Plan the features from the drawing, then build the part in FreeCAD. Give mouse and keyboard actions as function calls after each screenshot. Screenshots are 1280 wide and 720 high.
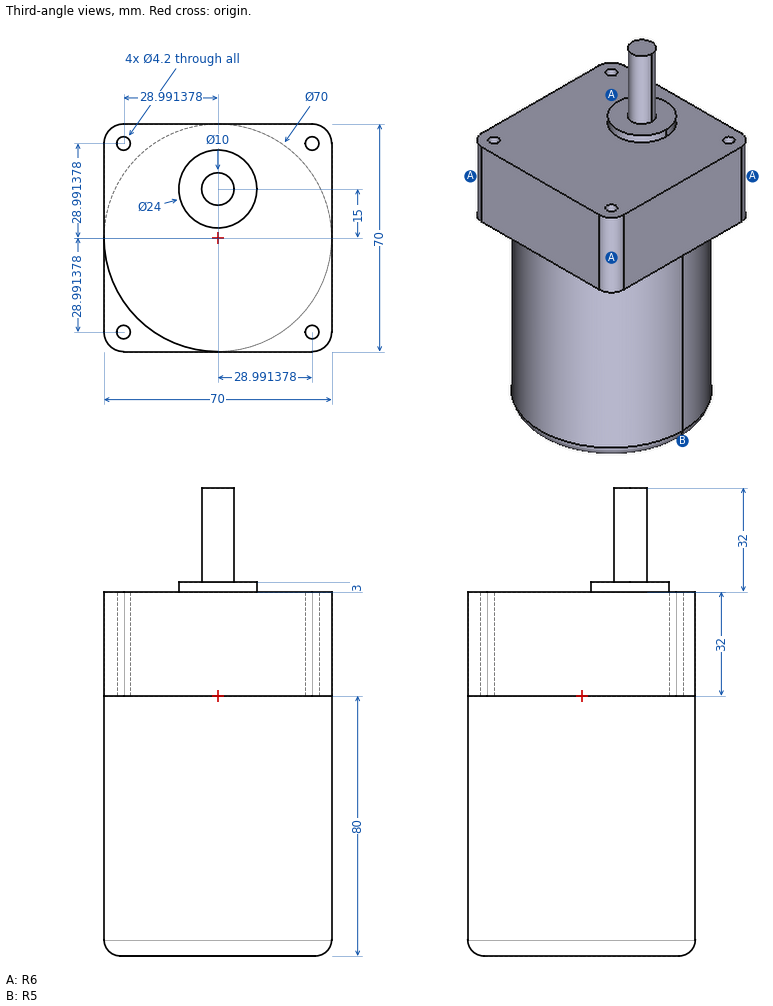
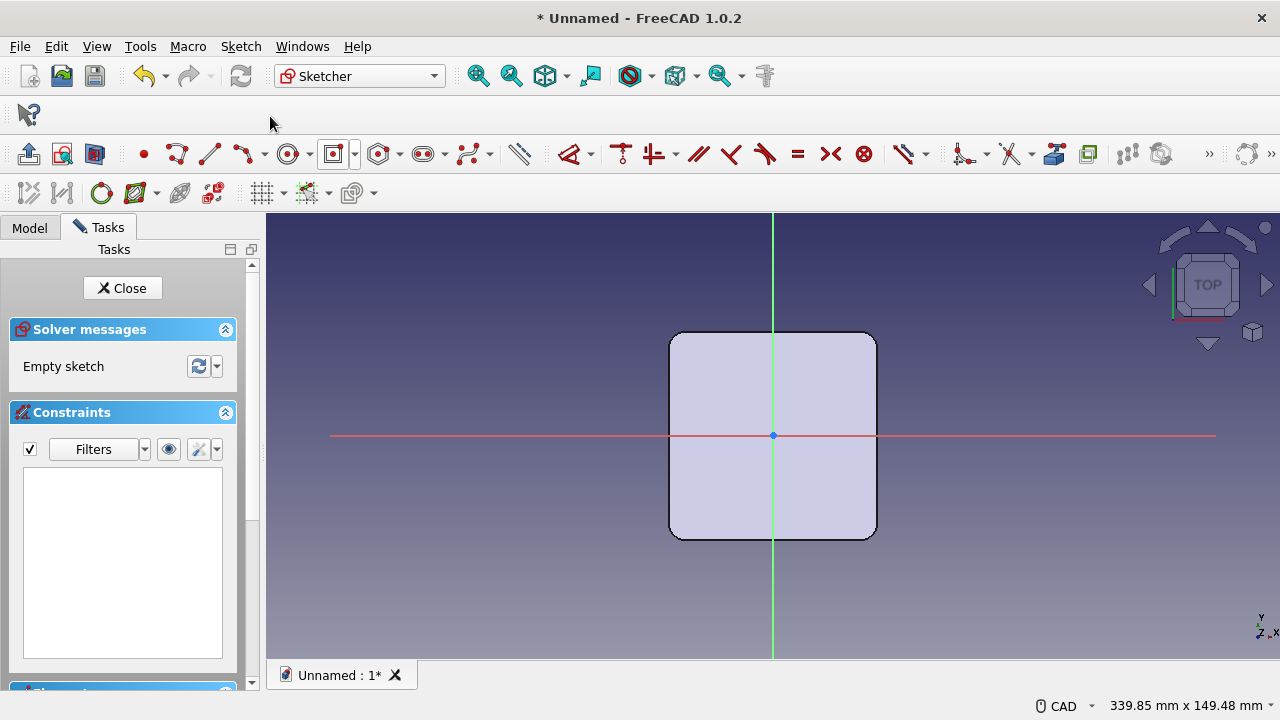
scroll(790, 399, up, 8)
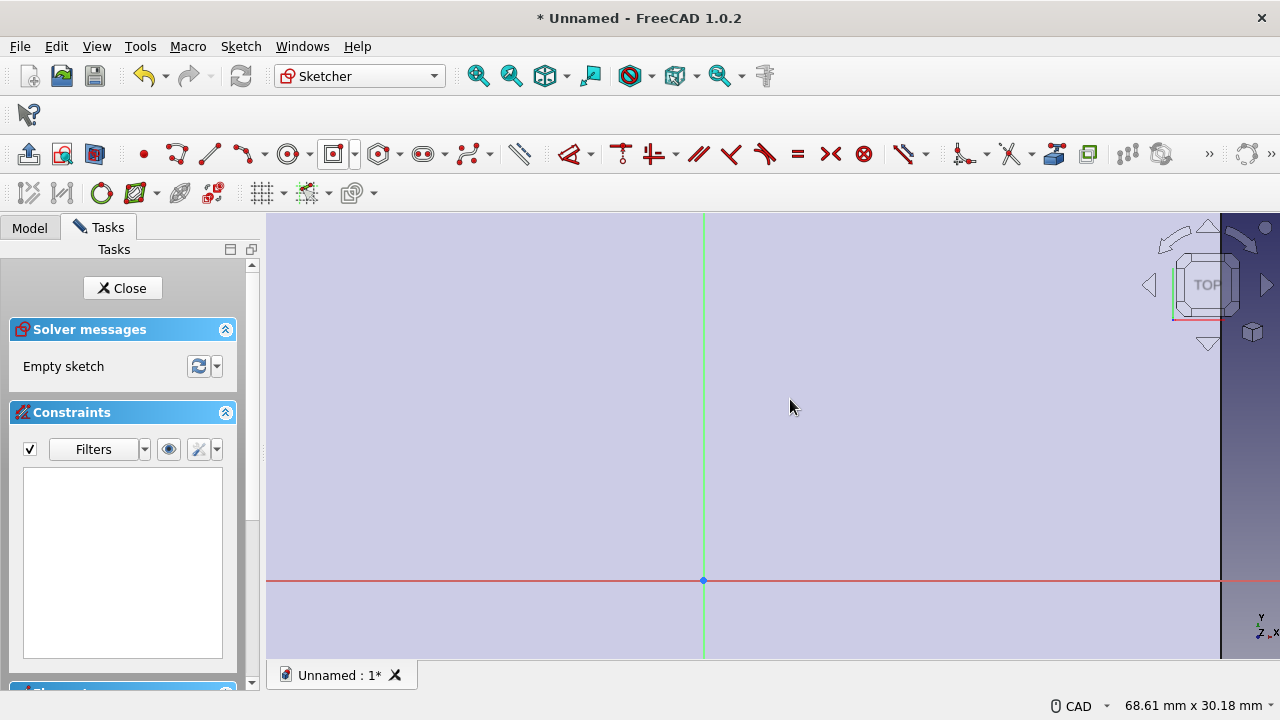
click(288, 154)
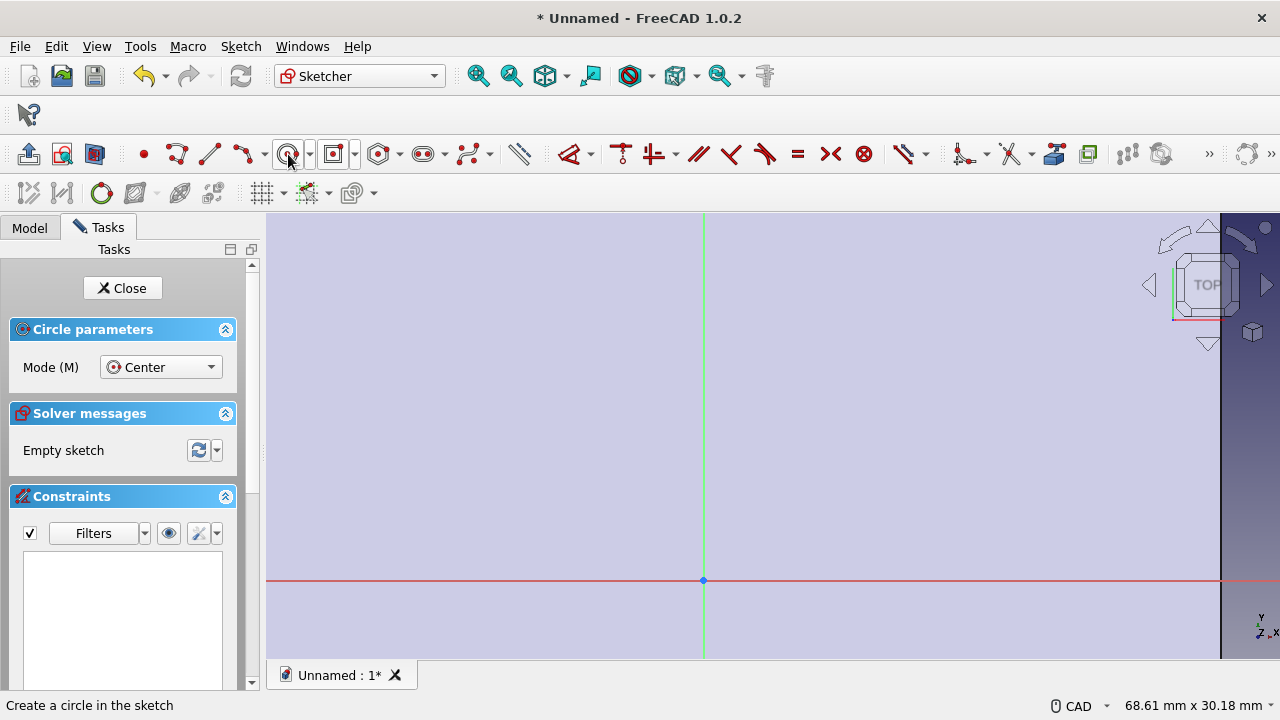
click(704, 359)
move(756, 307)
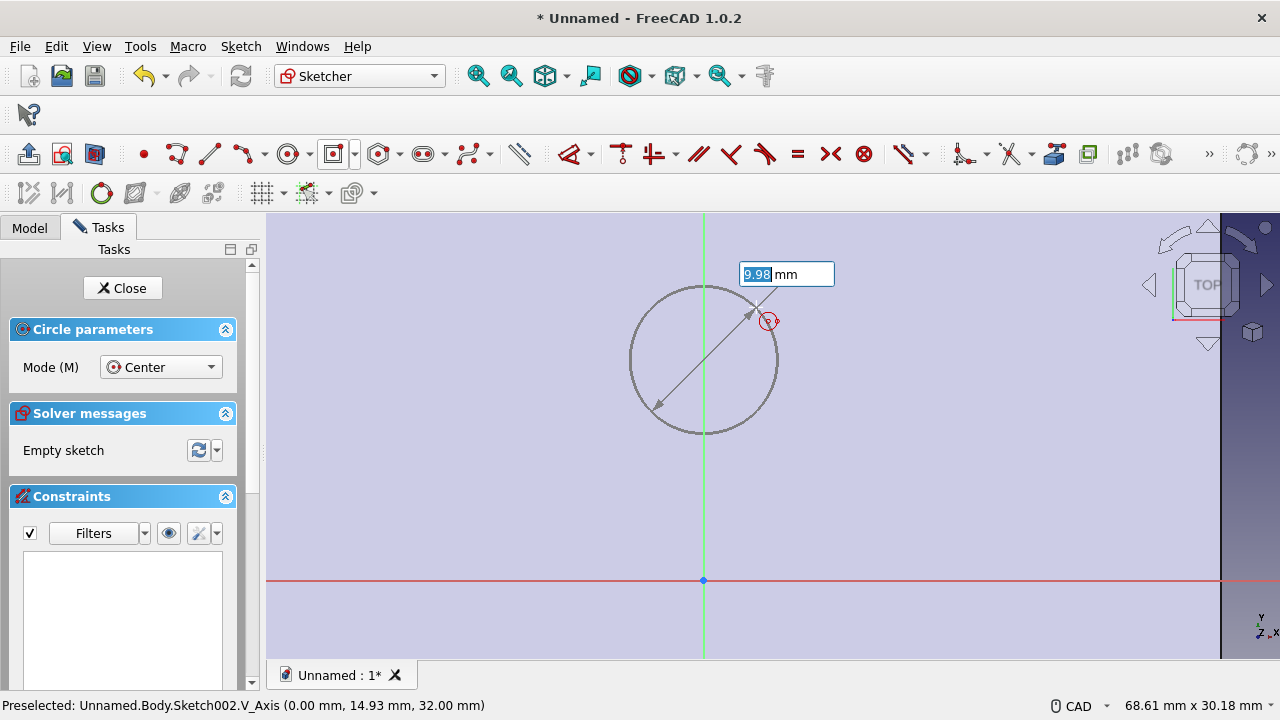
text(10)
key(Return)
key(Escape)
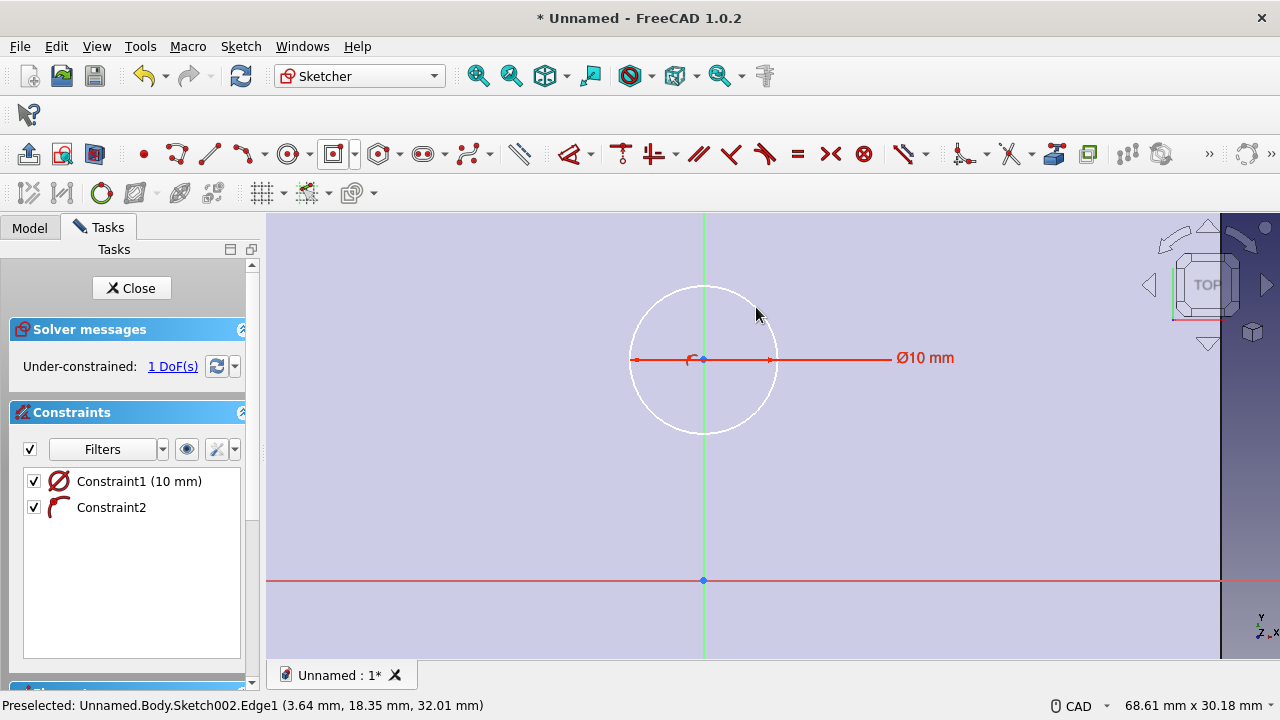
key(d)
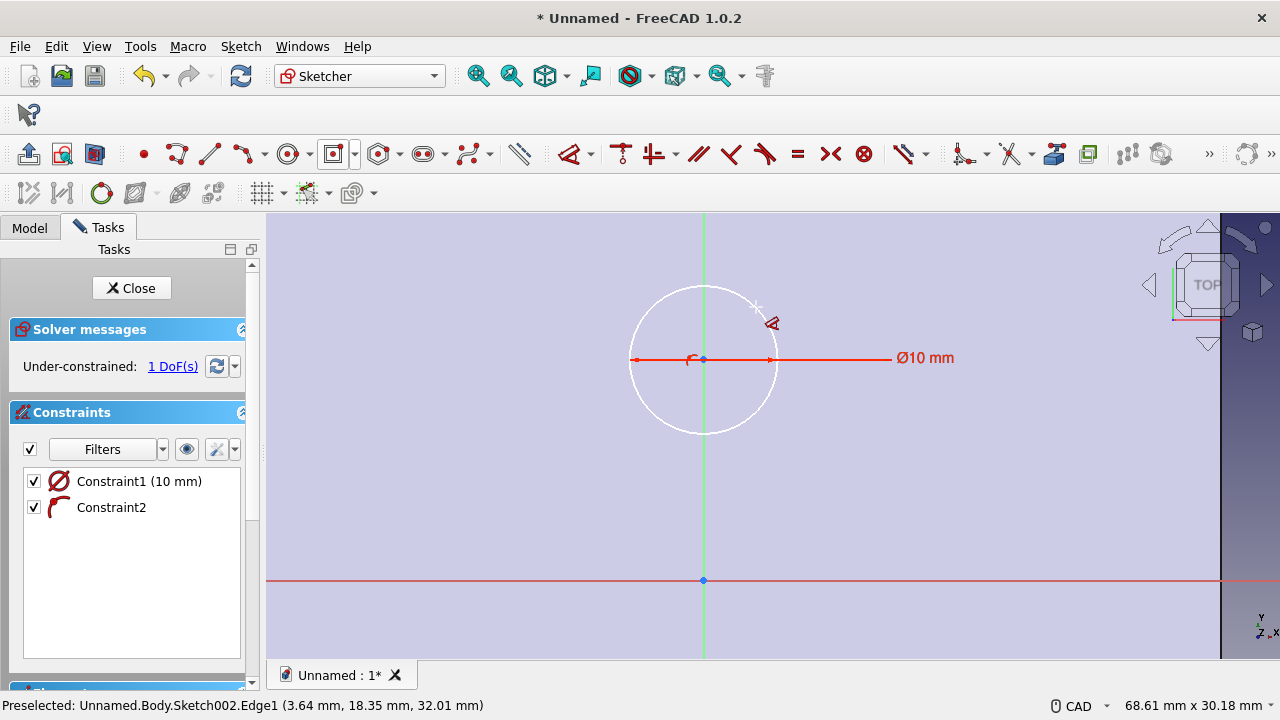
click(704, 360)
click(738, 470)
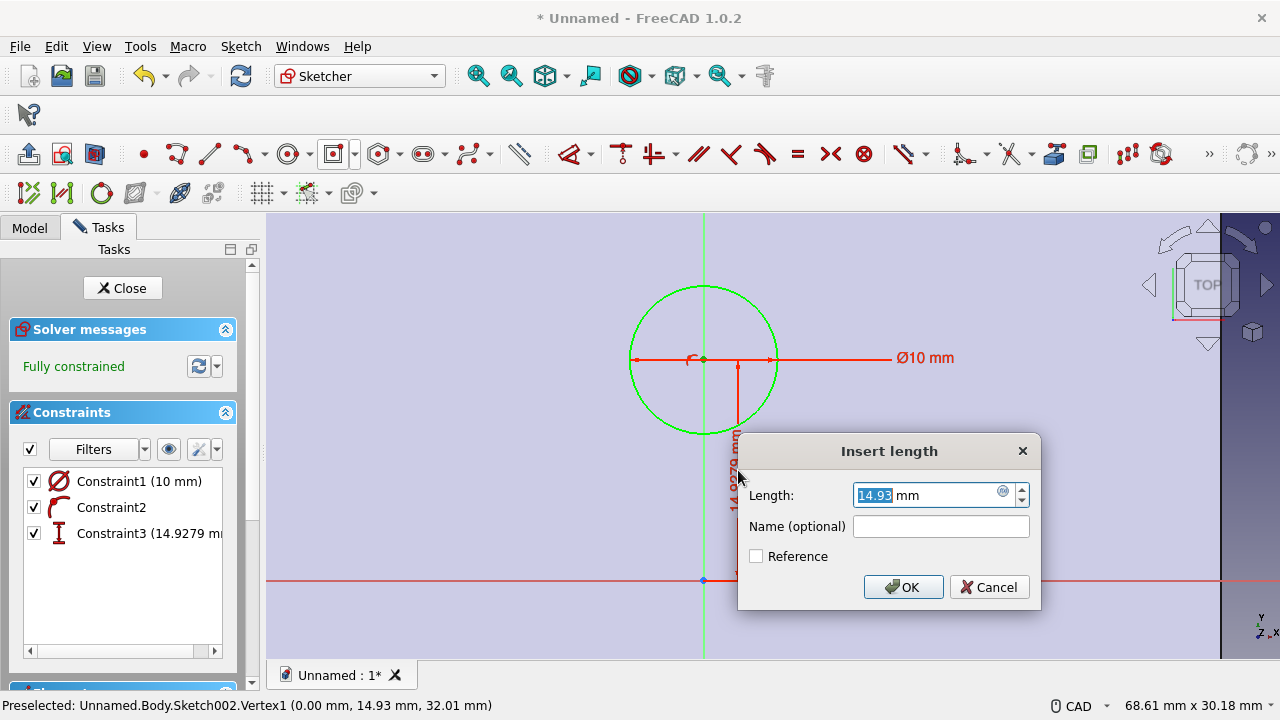
text(15)
key(Return)
key(Escape)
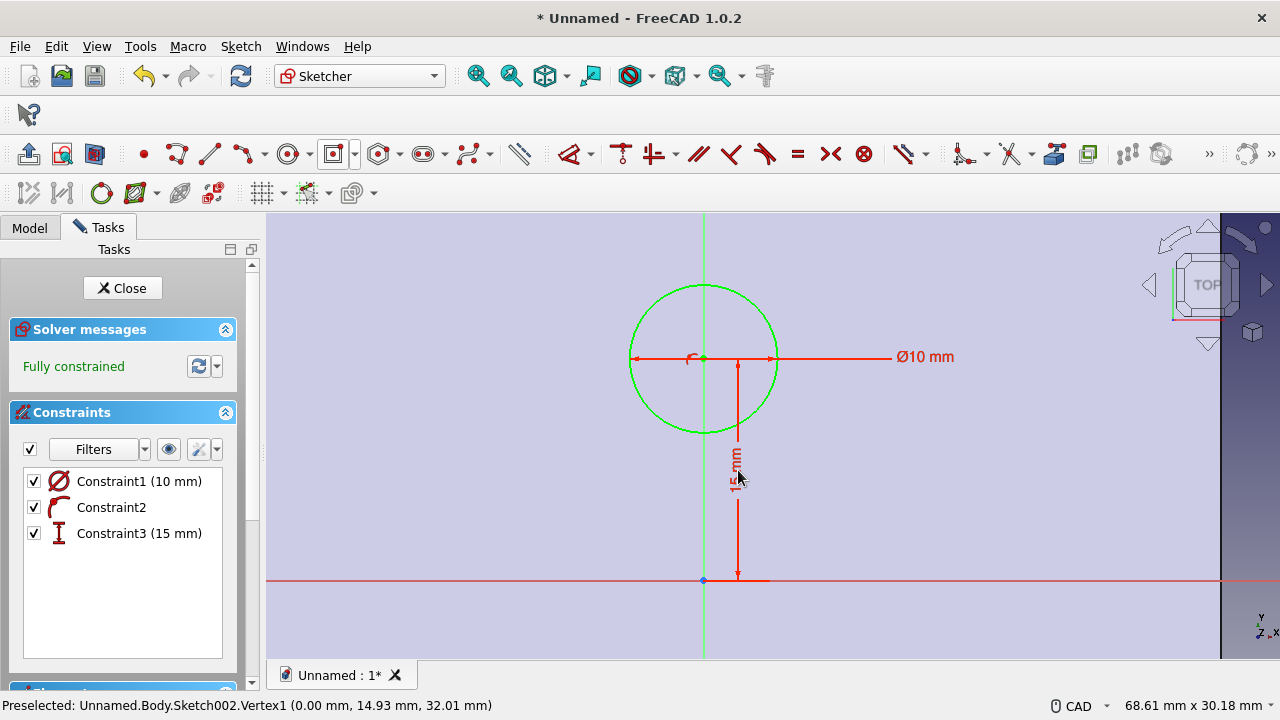
click(123, 288)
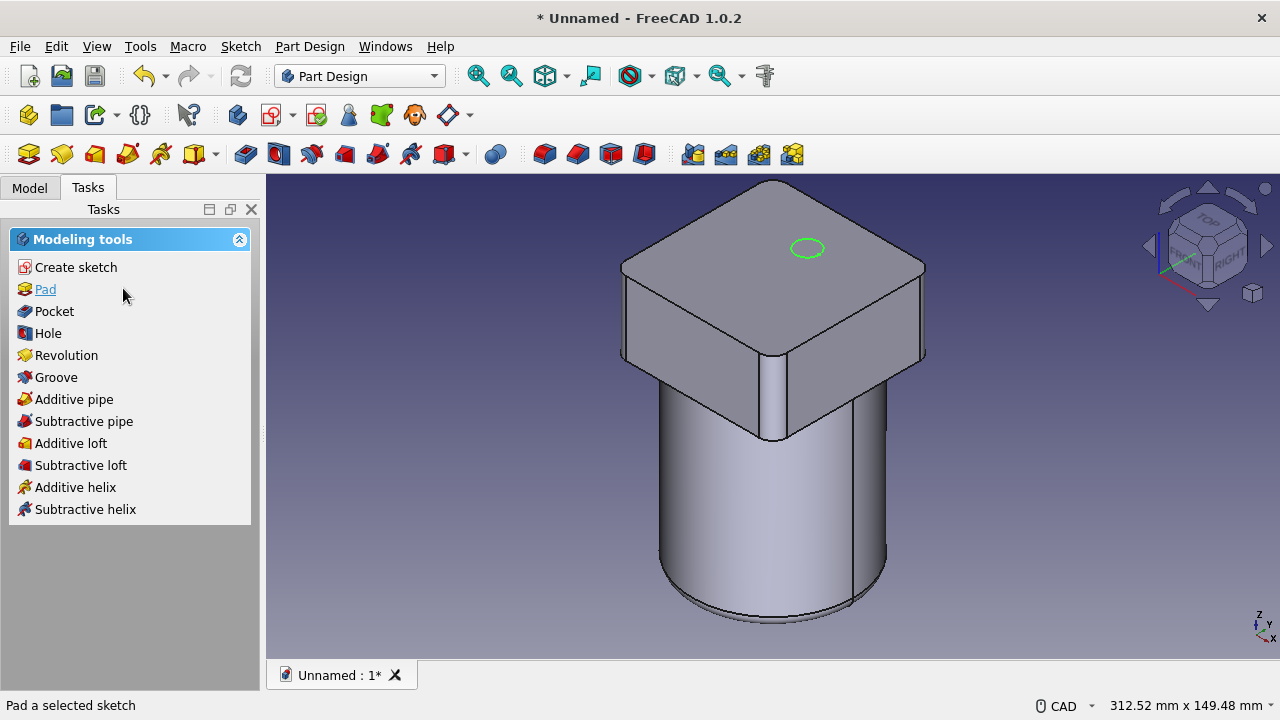
click(29, 154)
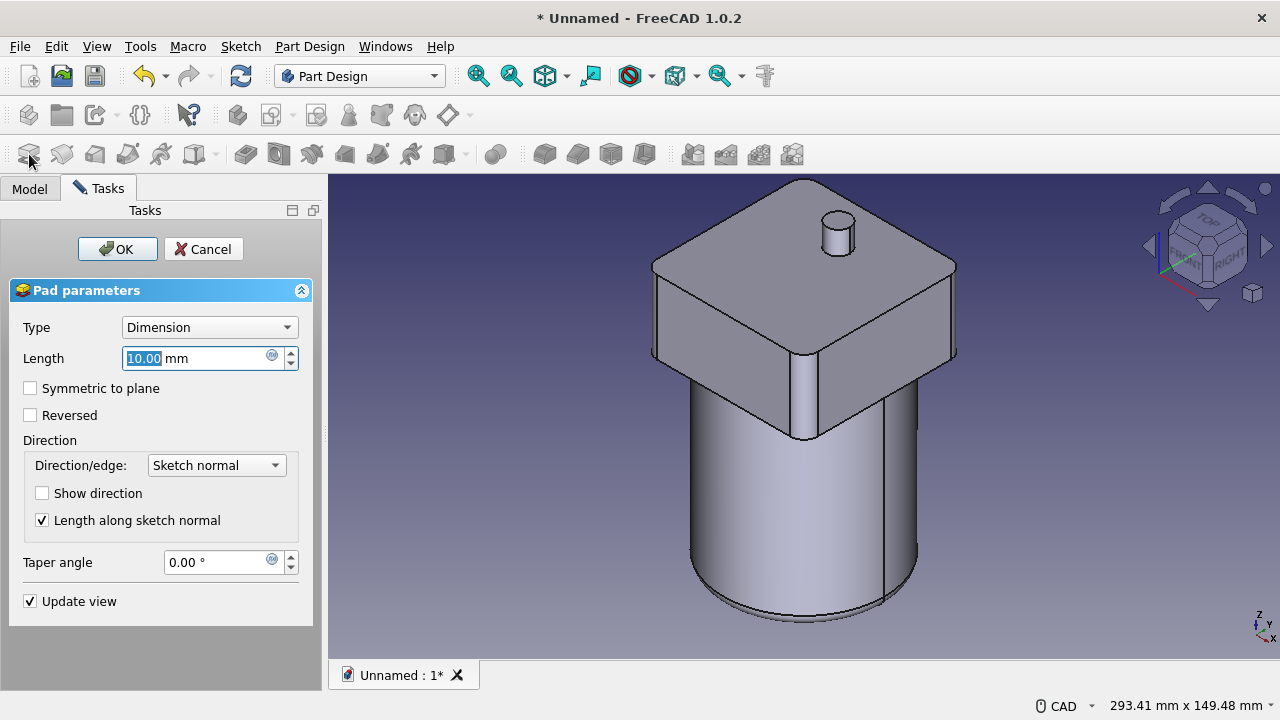
text(32)
key(Tab)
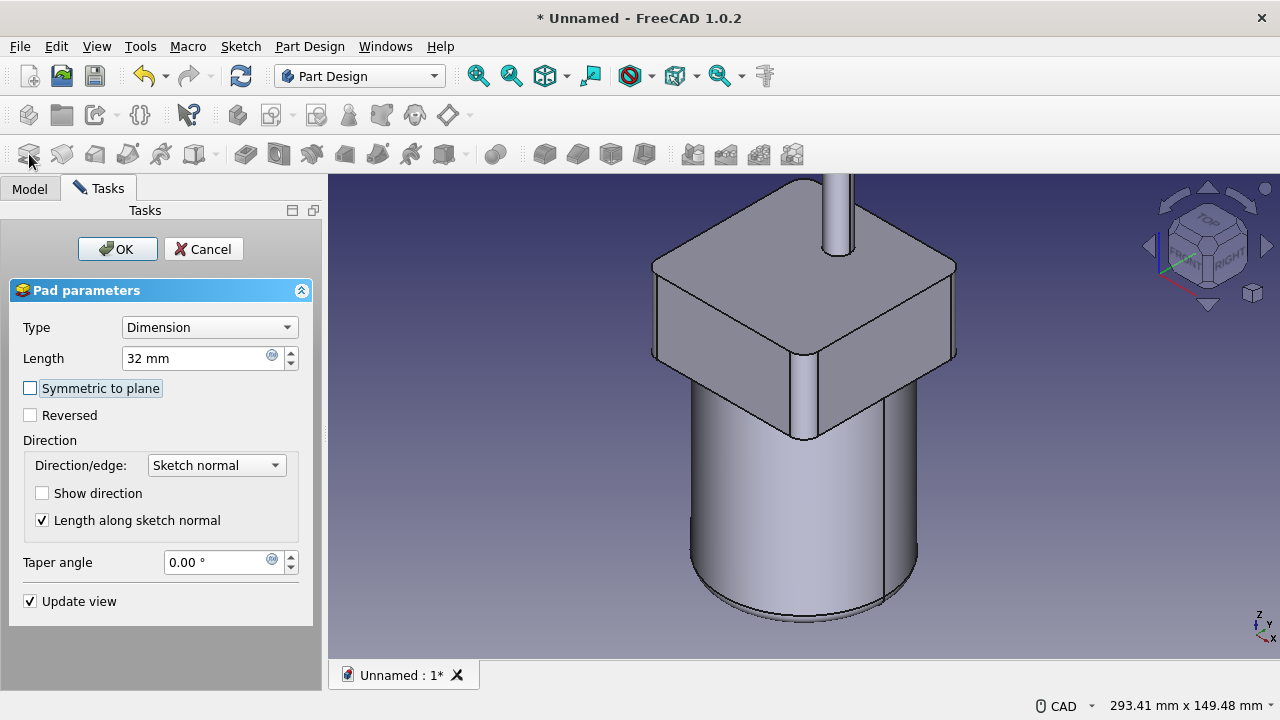
click(118, 249)